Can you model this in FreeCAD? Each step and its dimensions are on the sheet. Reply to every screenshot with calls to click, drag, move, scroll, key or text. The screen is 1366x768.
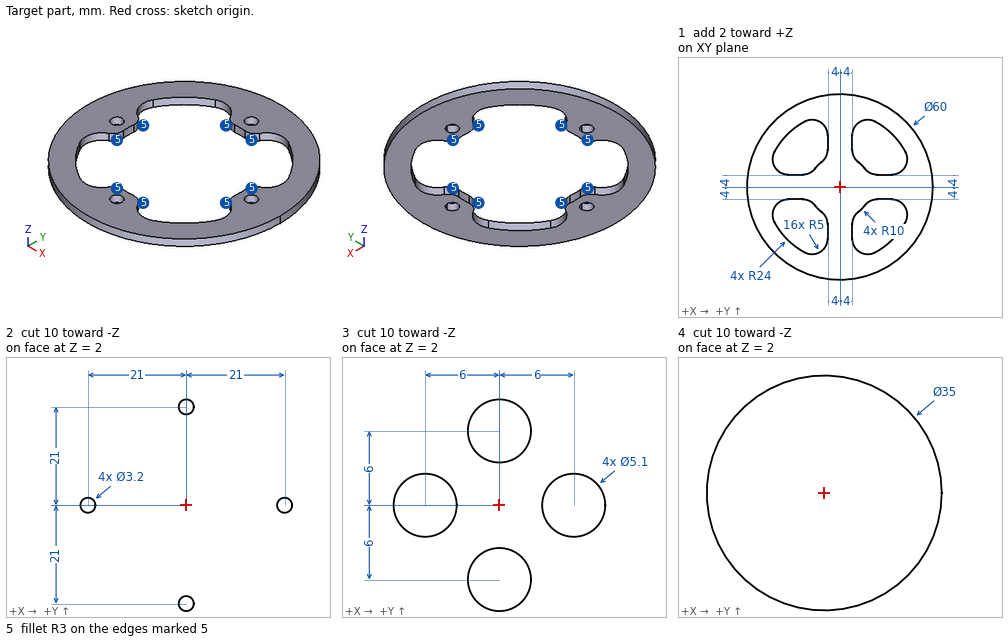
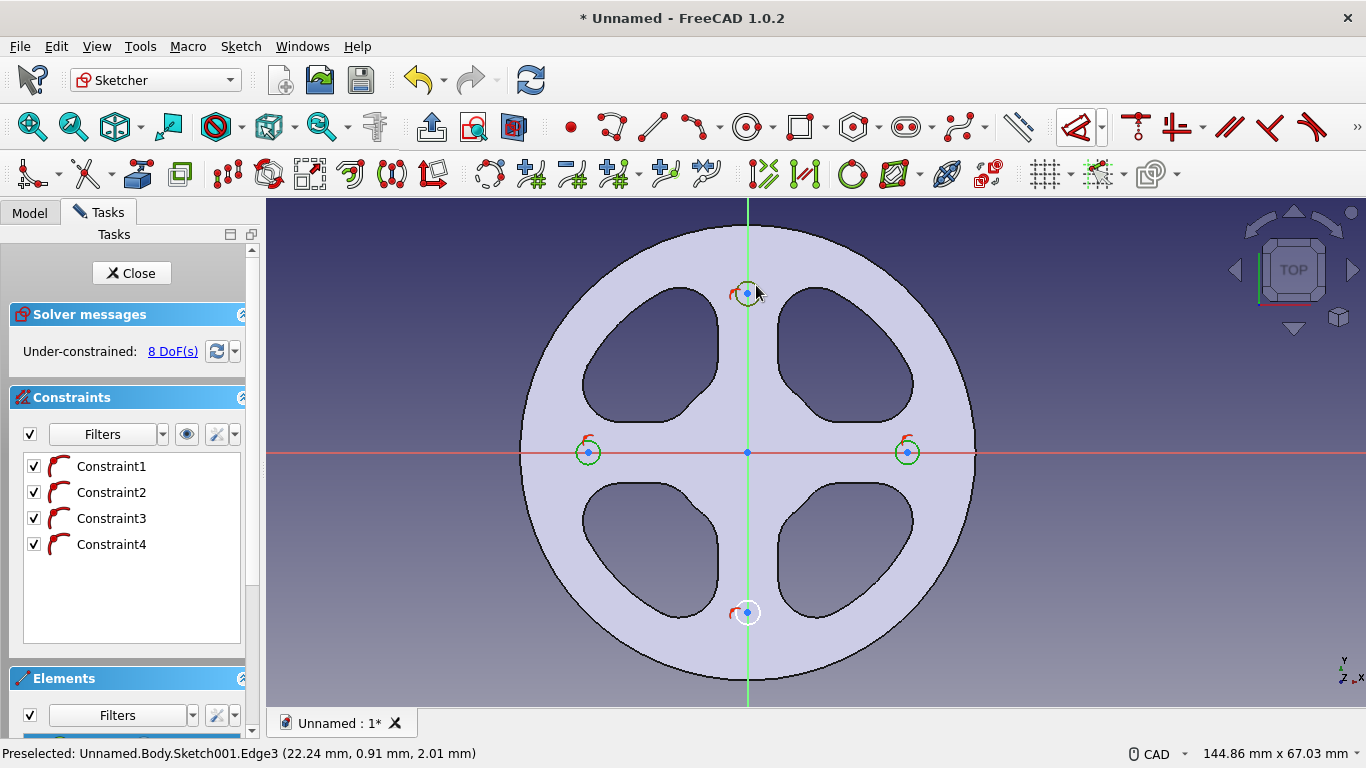
scroll(756, 604, up, 3)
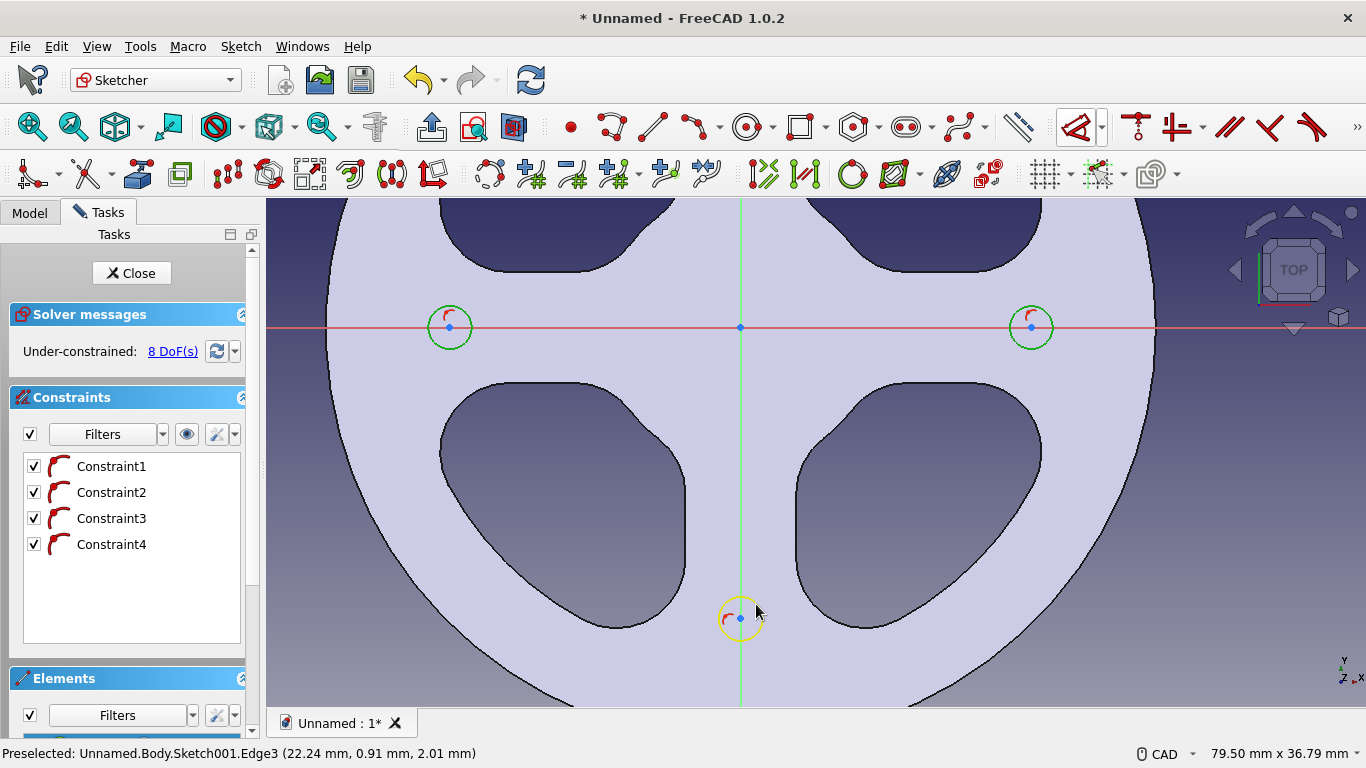
click(756, 603)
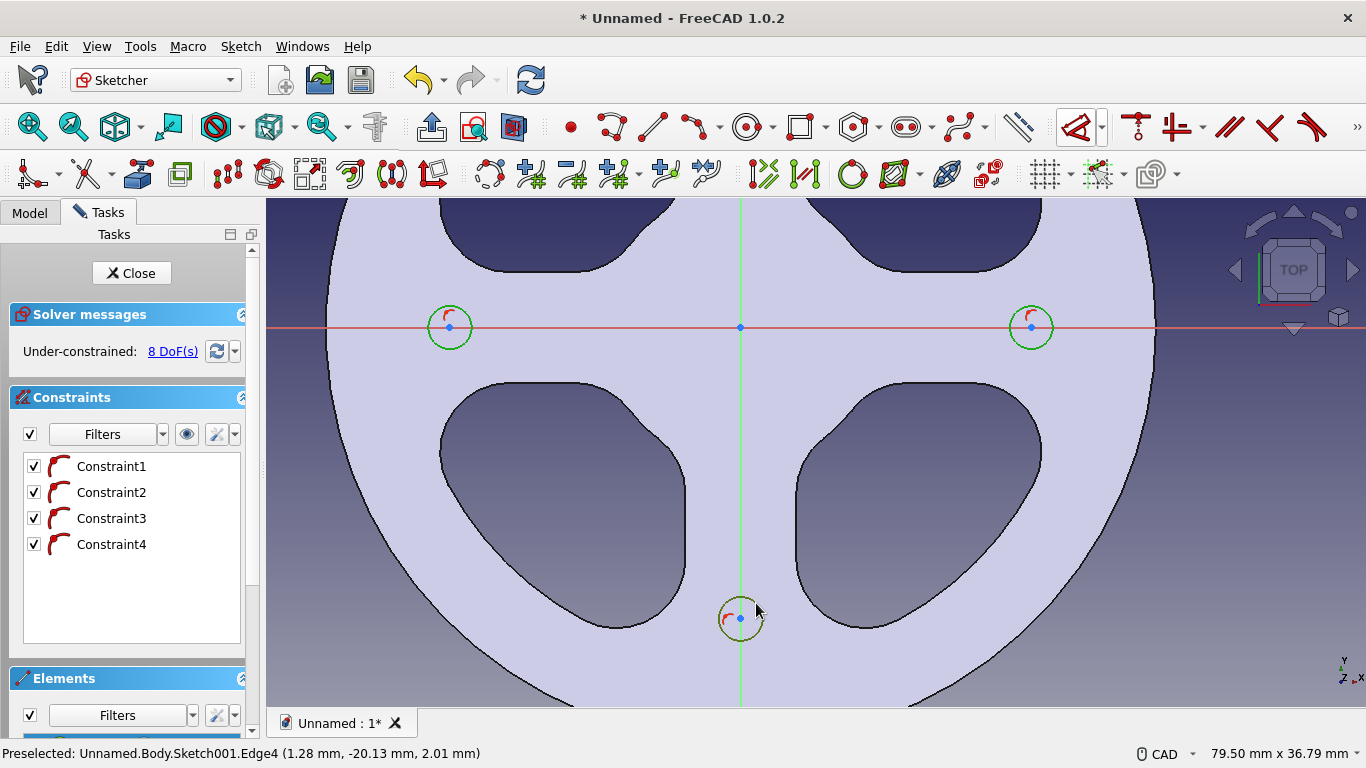
key(e)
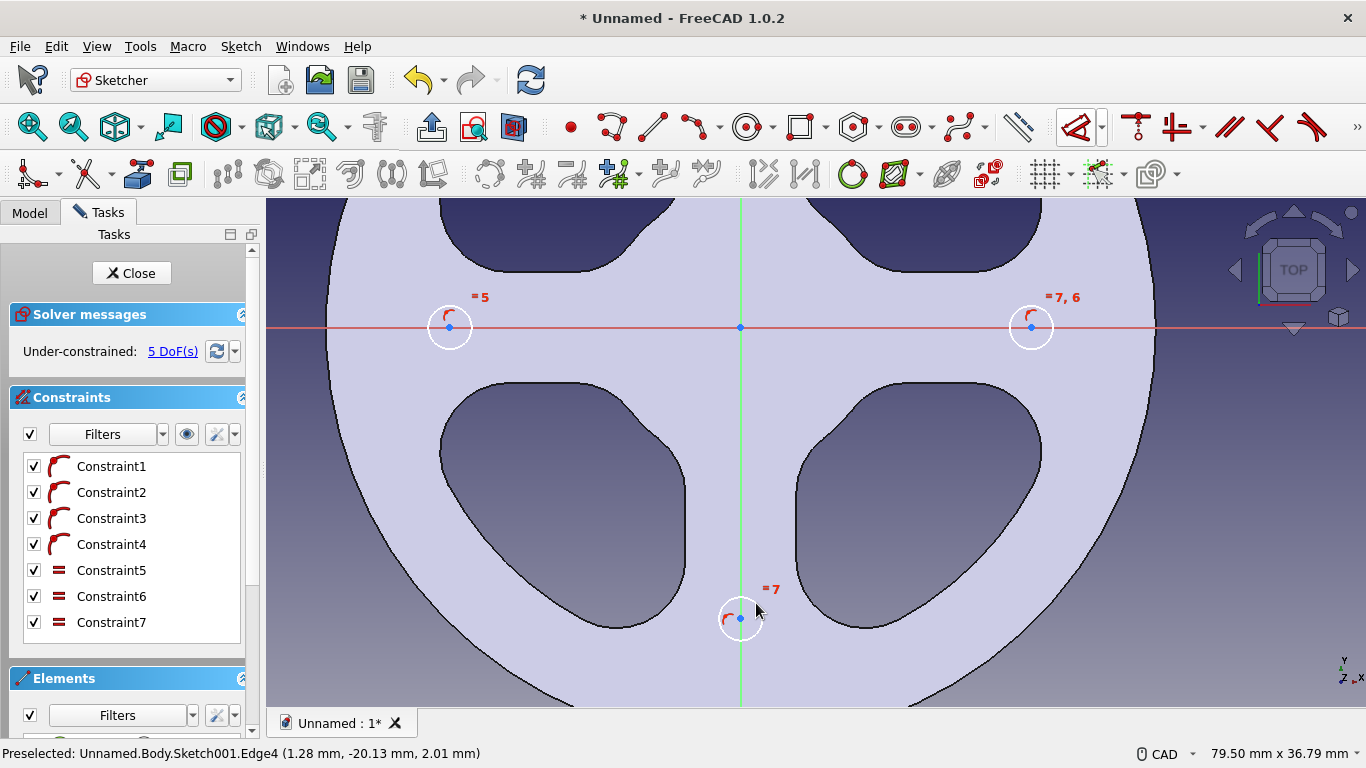
click(1076, 128)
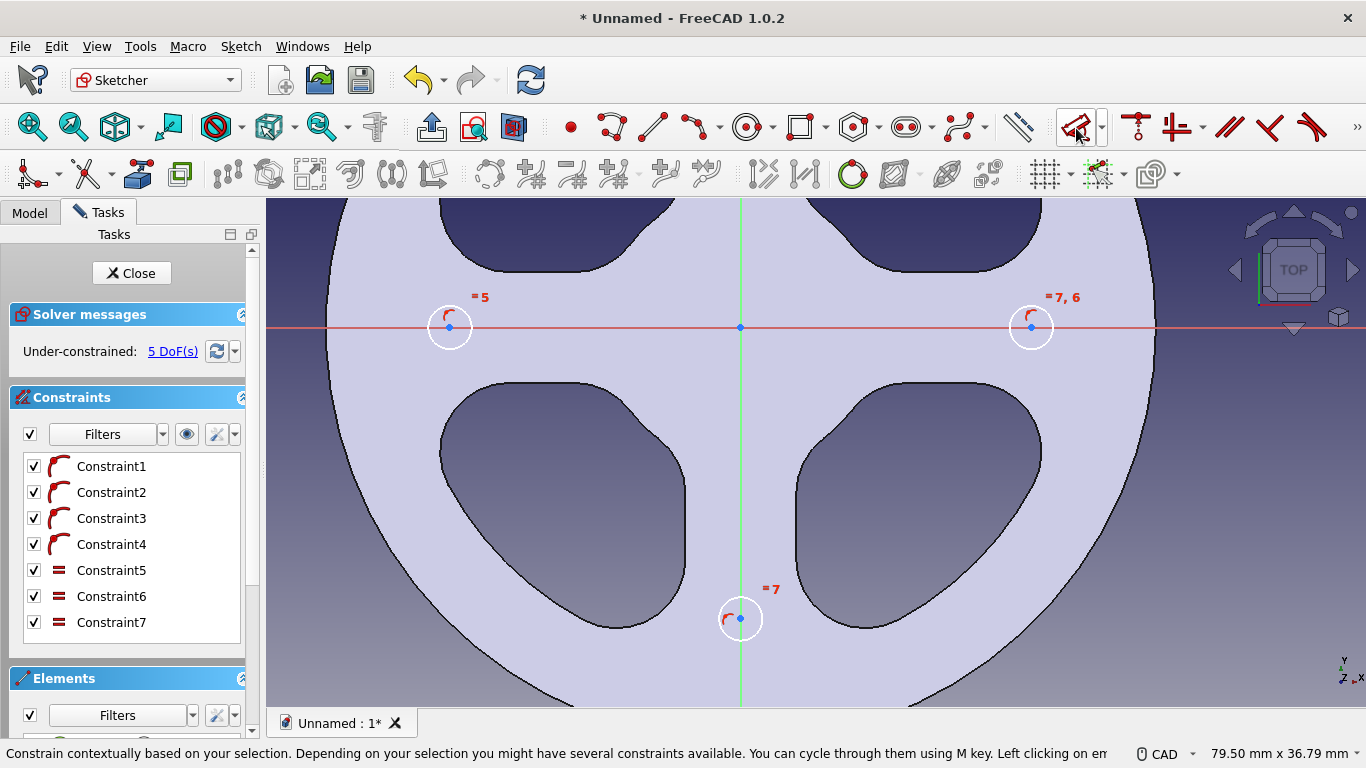
click(465, 312)
click(487, 289)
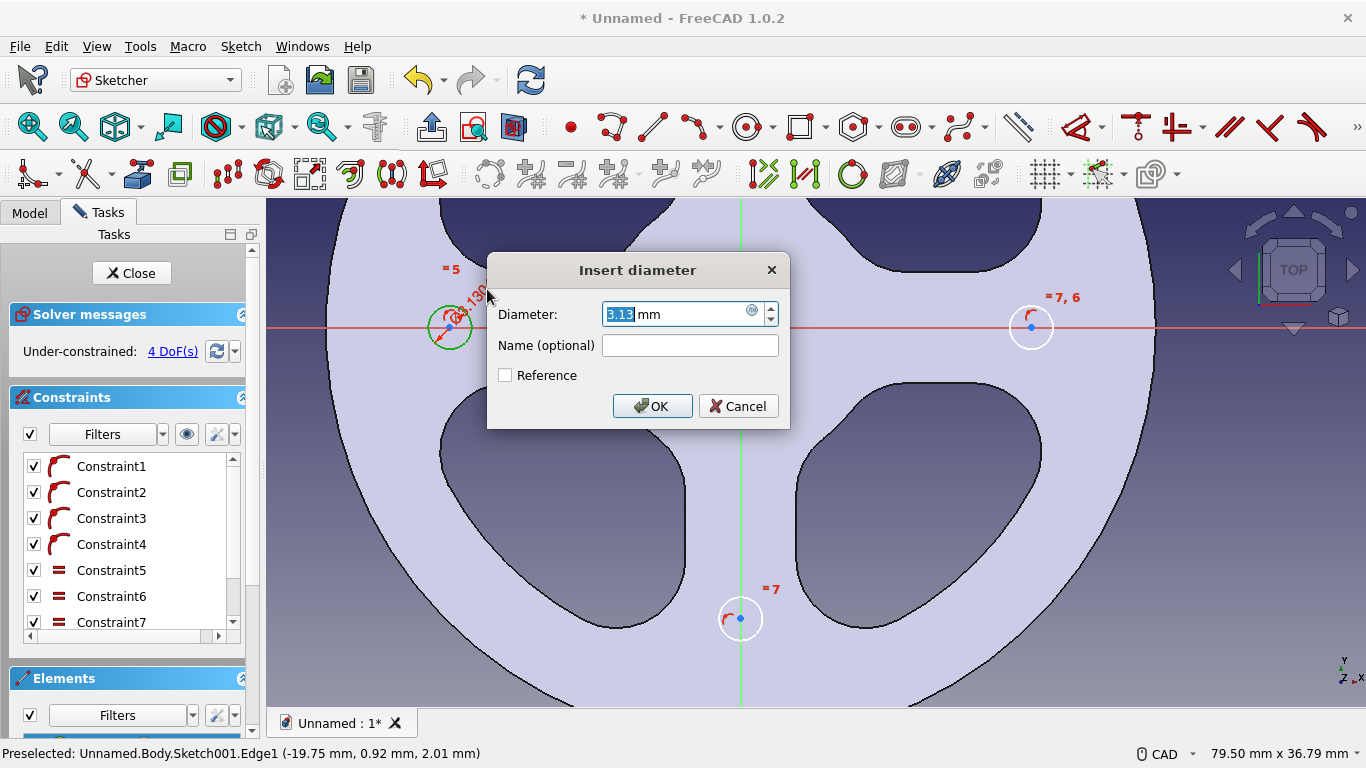
text(3.2)
key(Return)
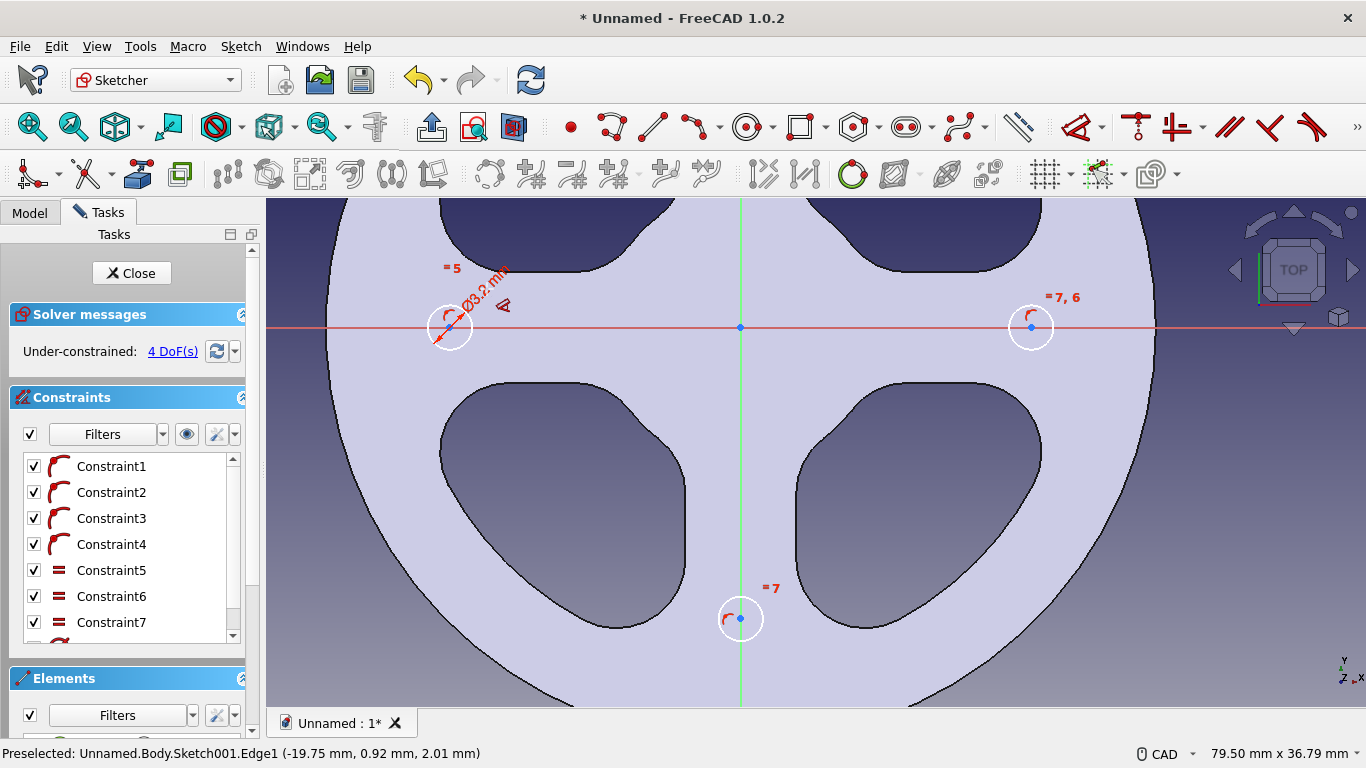
click(450, 328)
click(595, 362)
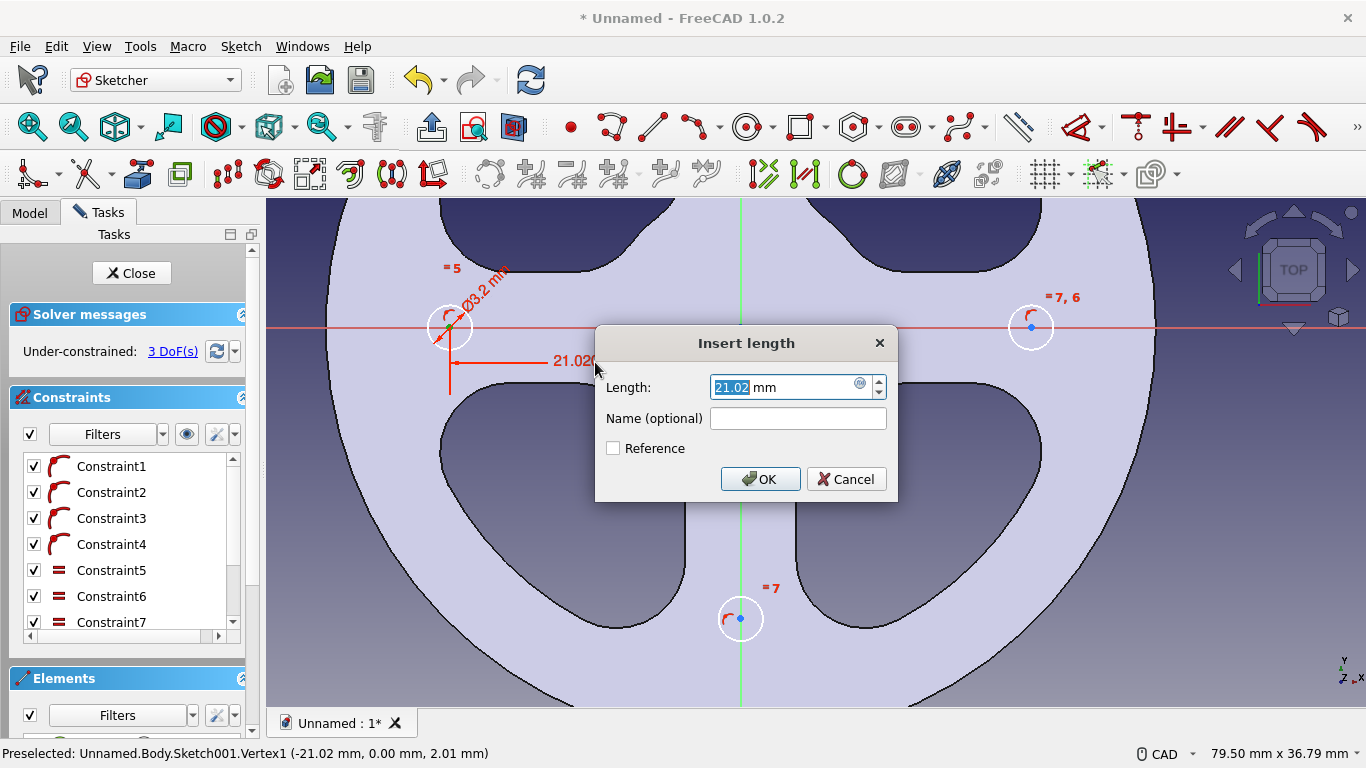
text(21)
key(Return)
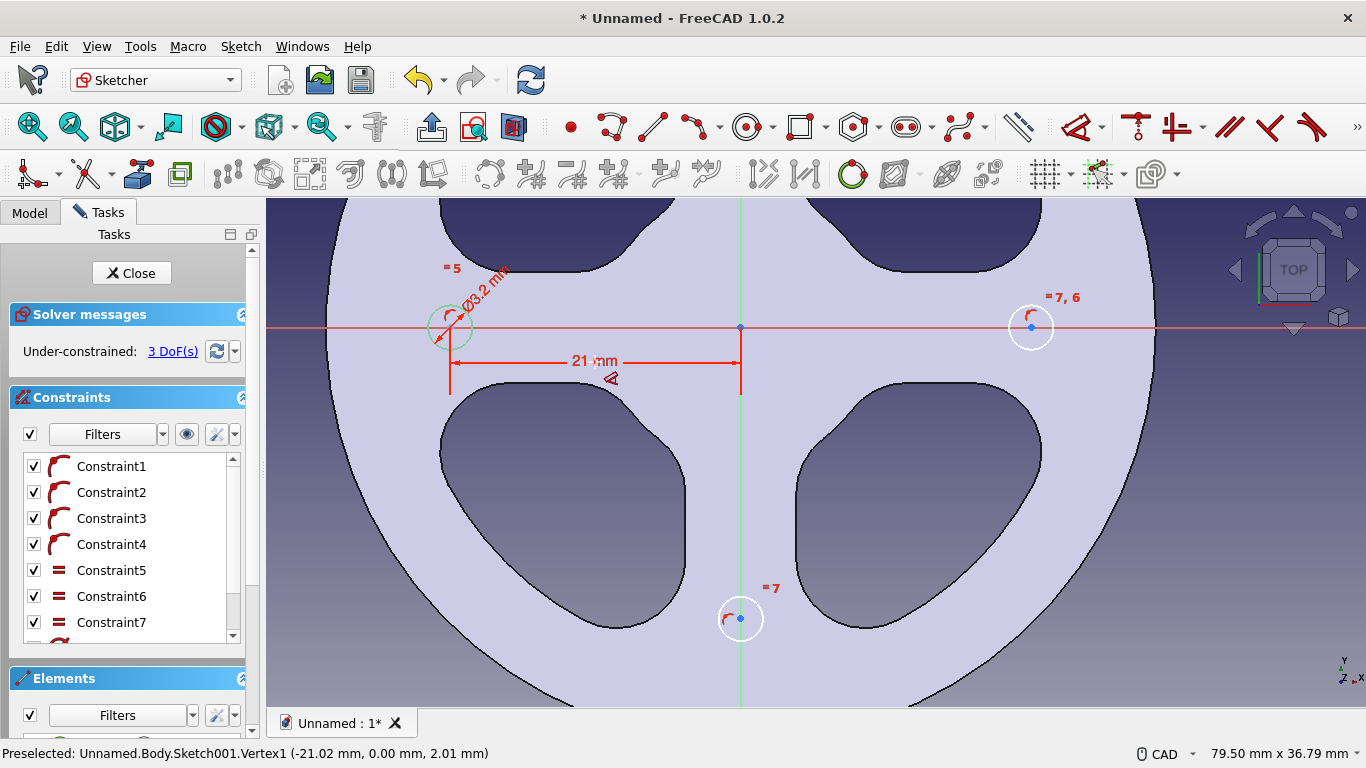
scroll(756, 604, down, 3)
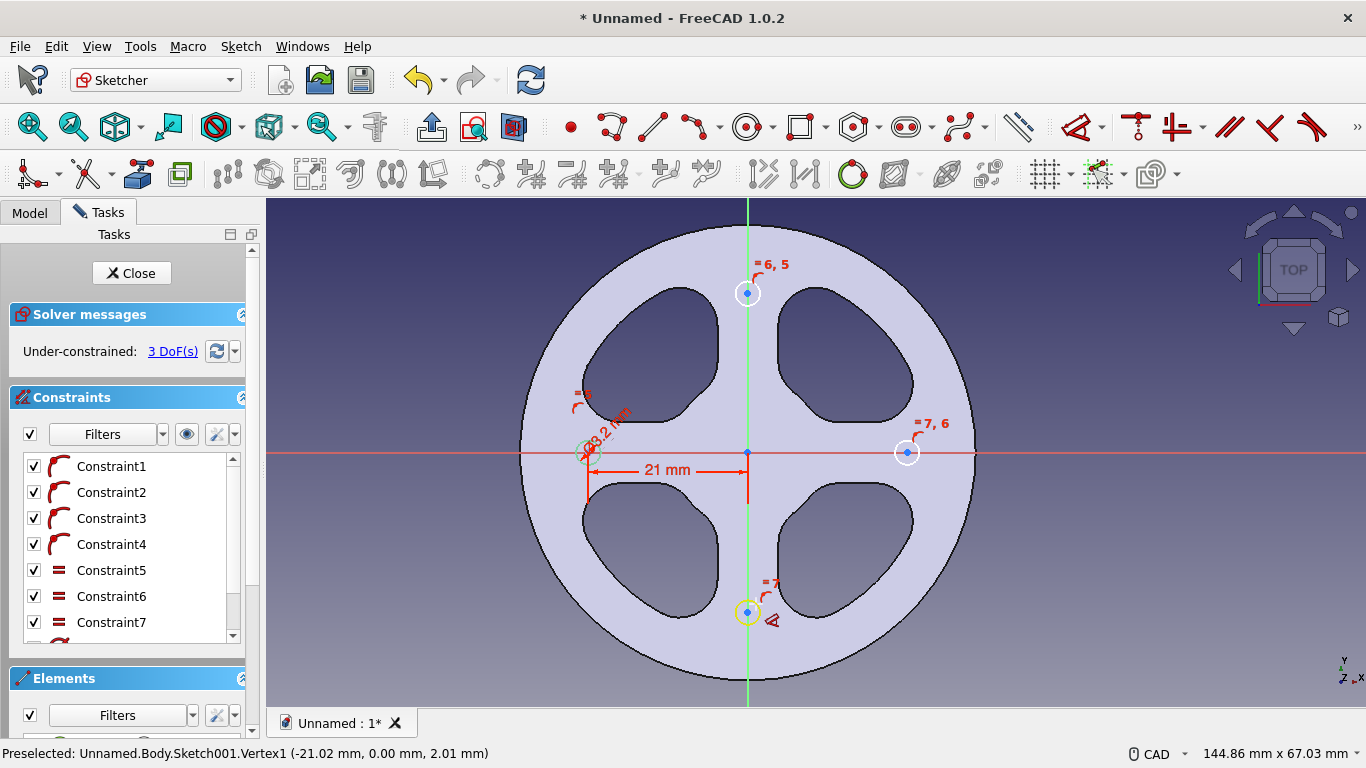
click(748, 294)
click(782, 373)